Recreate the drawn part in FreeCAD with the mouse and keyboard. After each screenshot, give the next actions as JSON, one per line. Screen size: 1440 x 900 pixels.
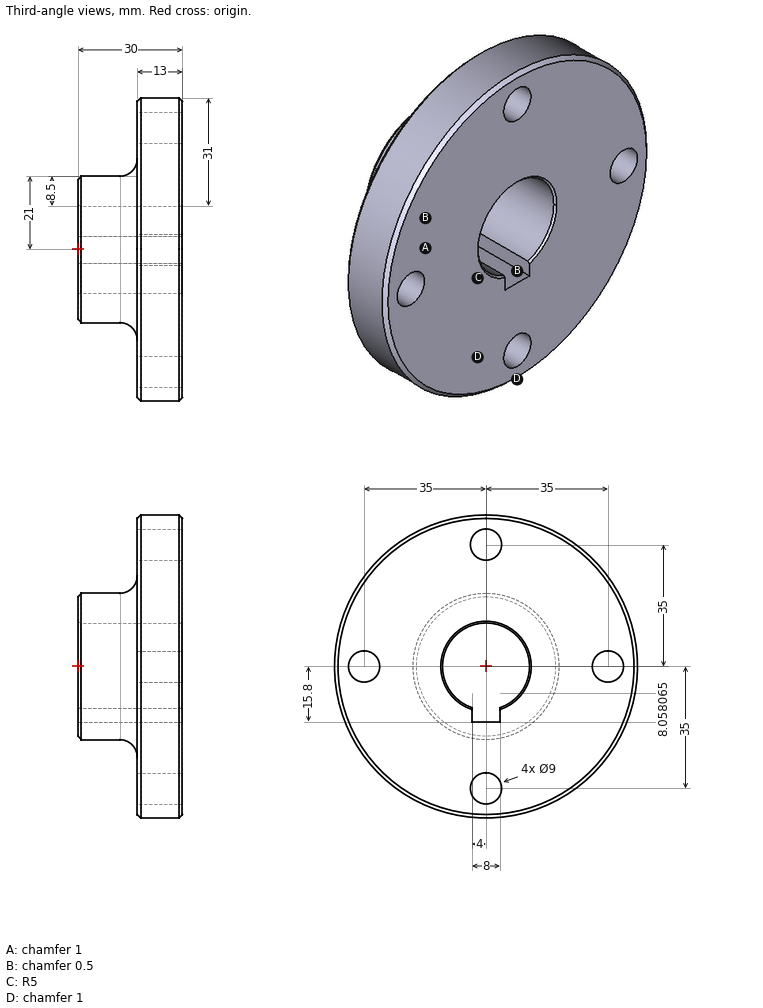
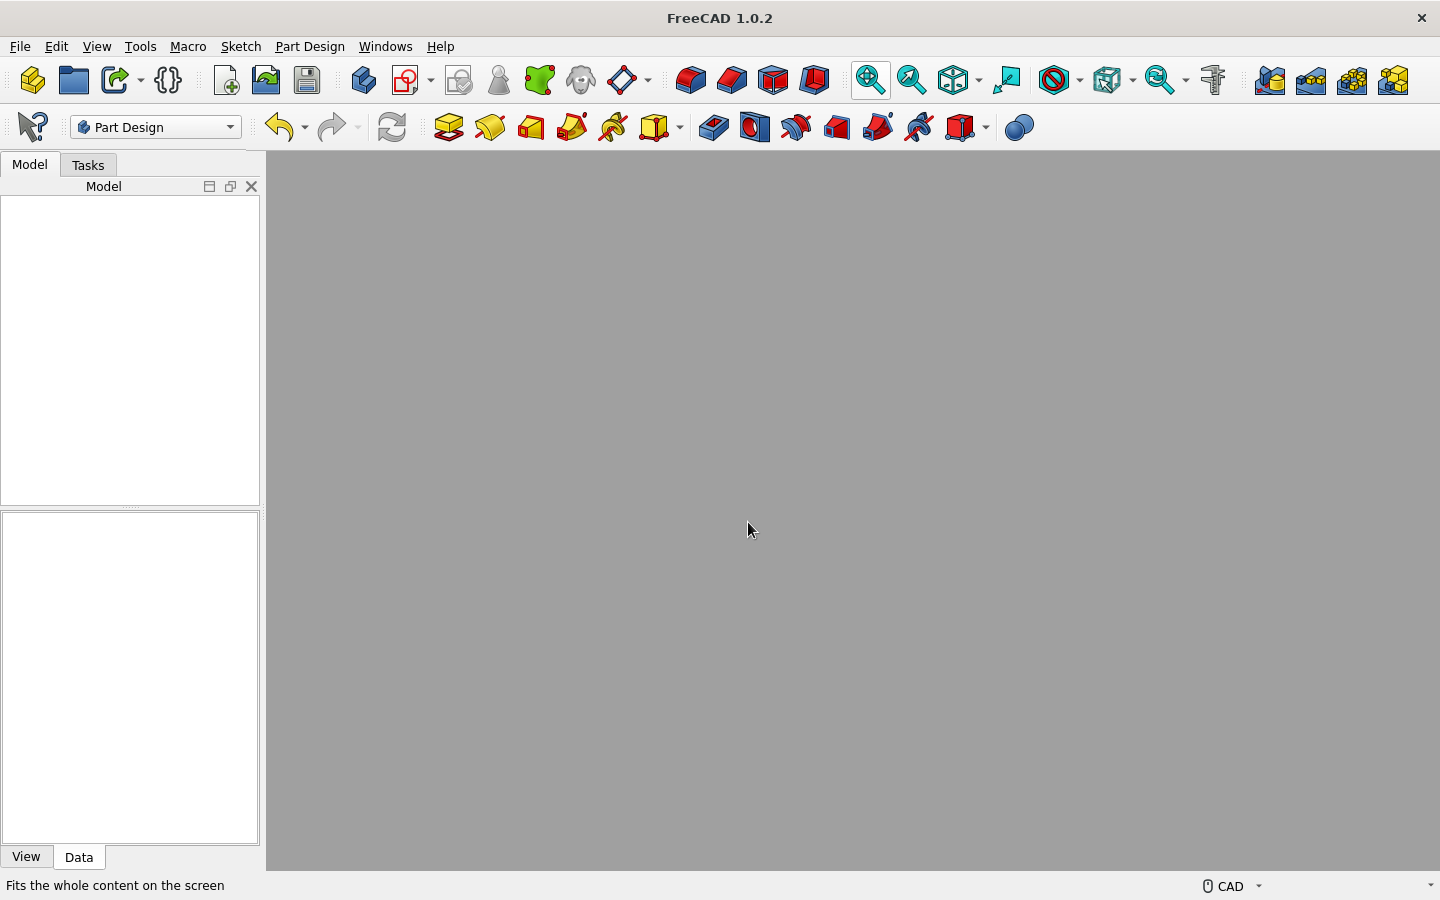
{"action": "left_click", "coordinate": [225, 80]}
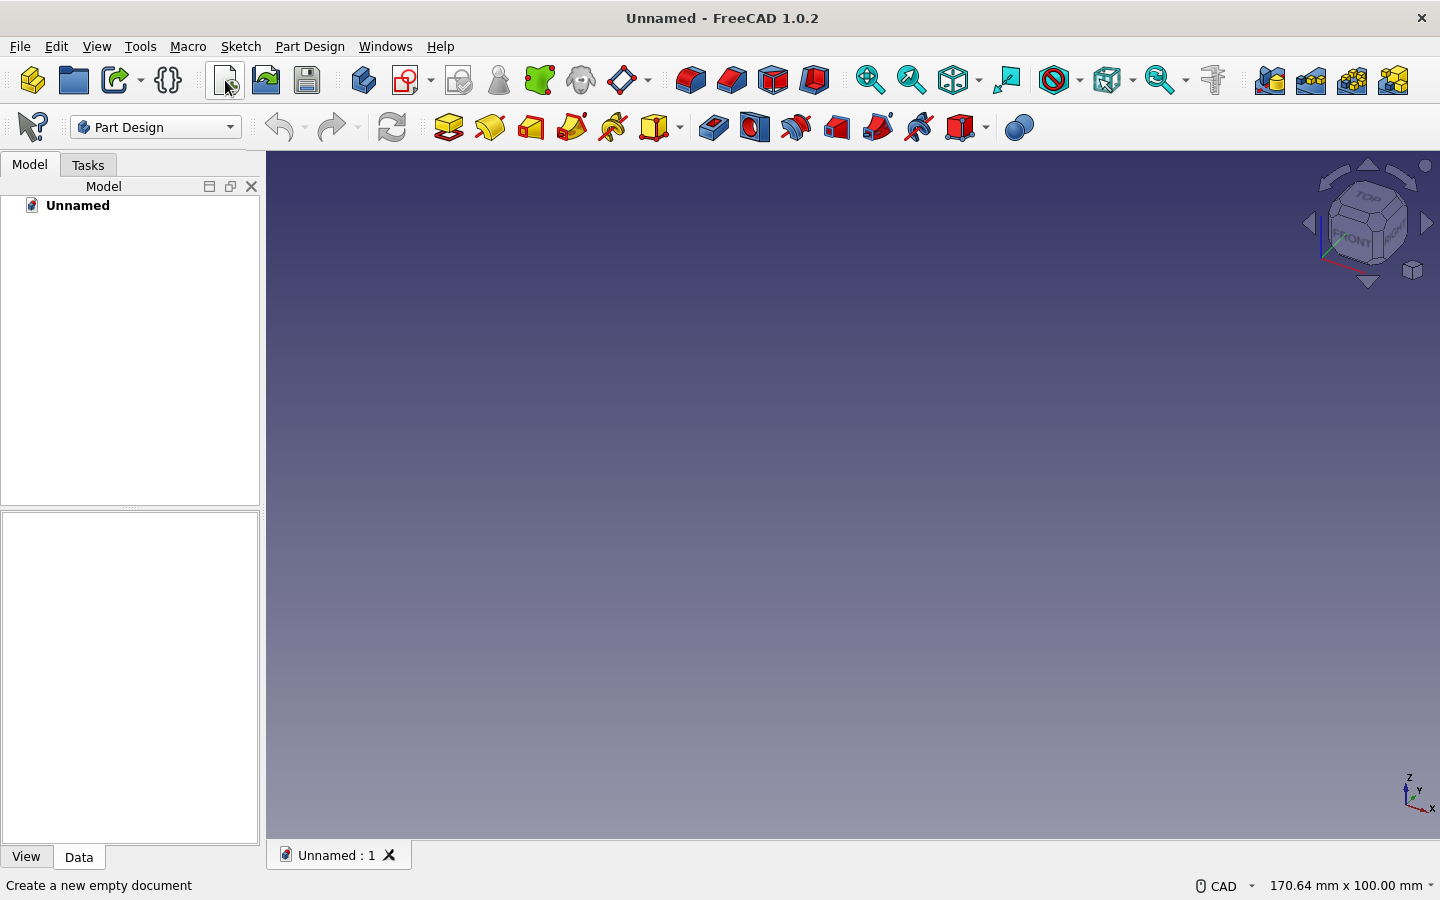
{"action": "left_click", "coordinate": [404, 80]}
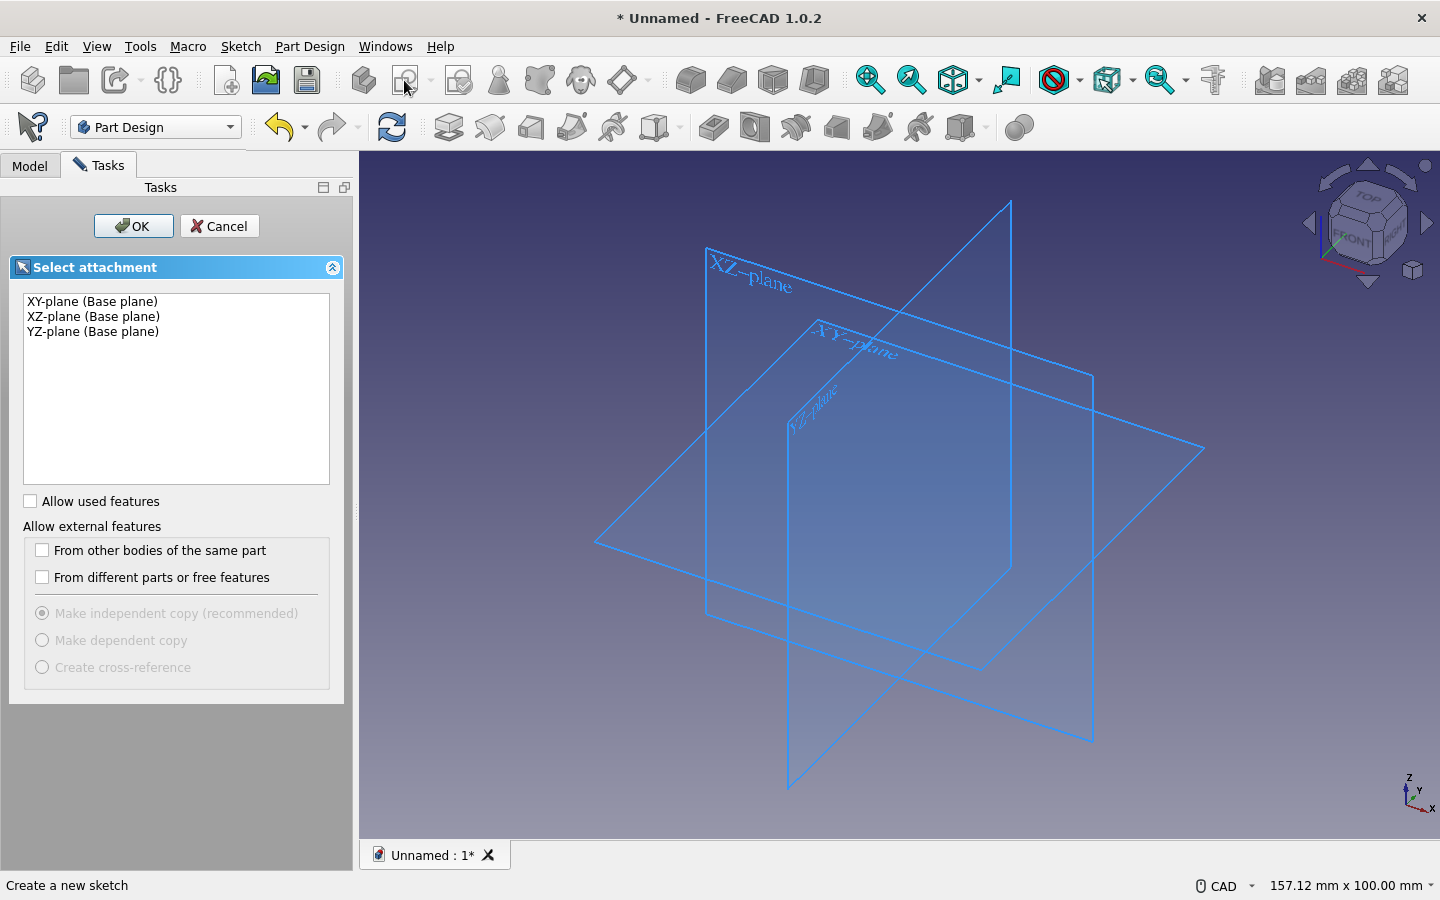
{"action": "left_click", "coordinate": [84, 302]}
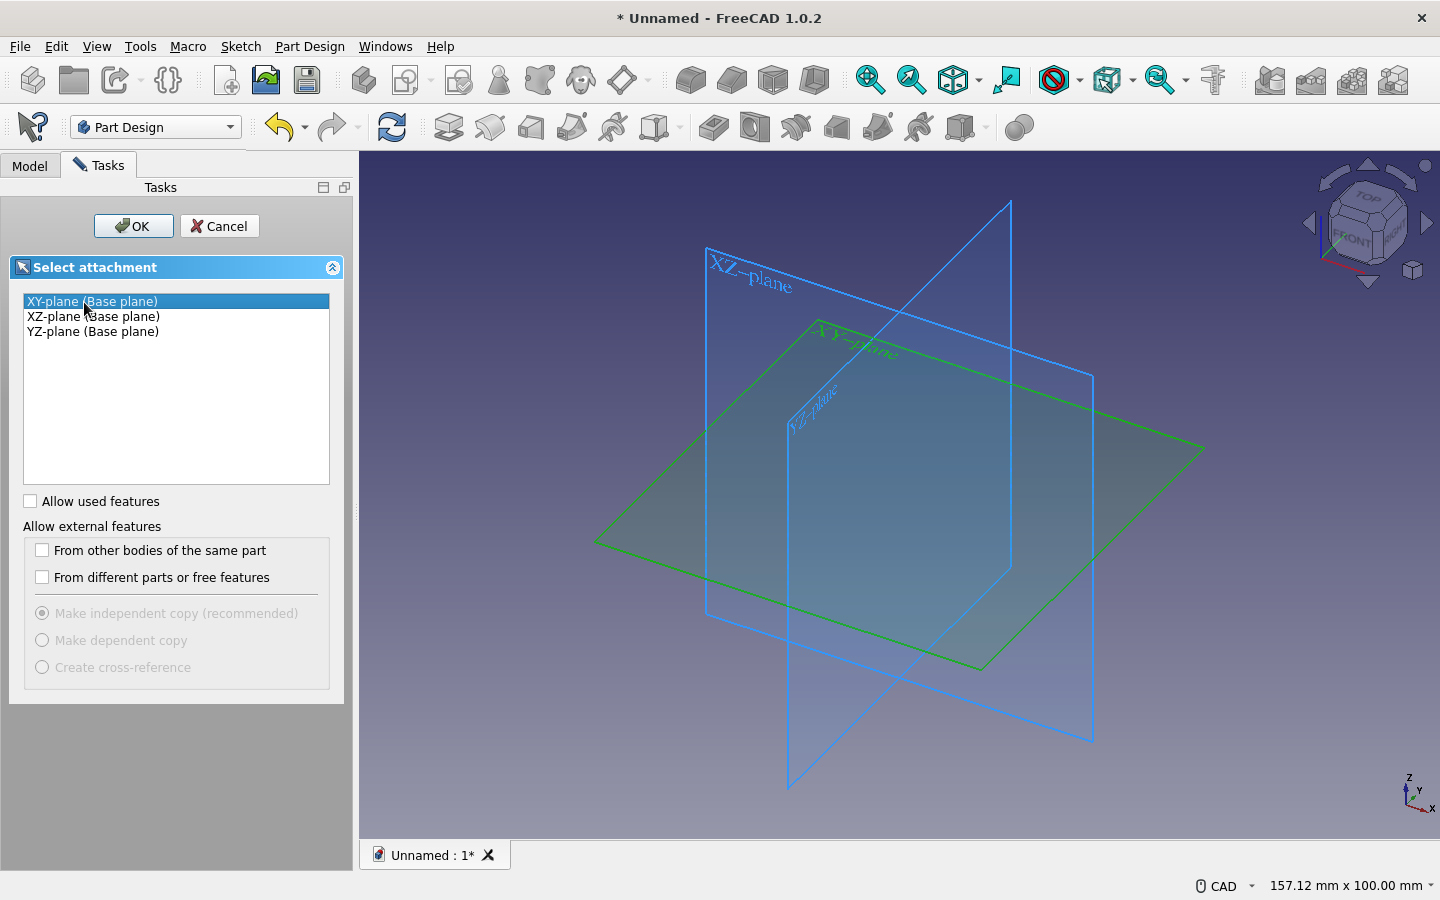
{"action": "left_click", "coordinate": [134, 226]}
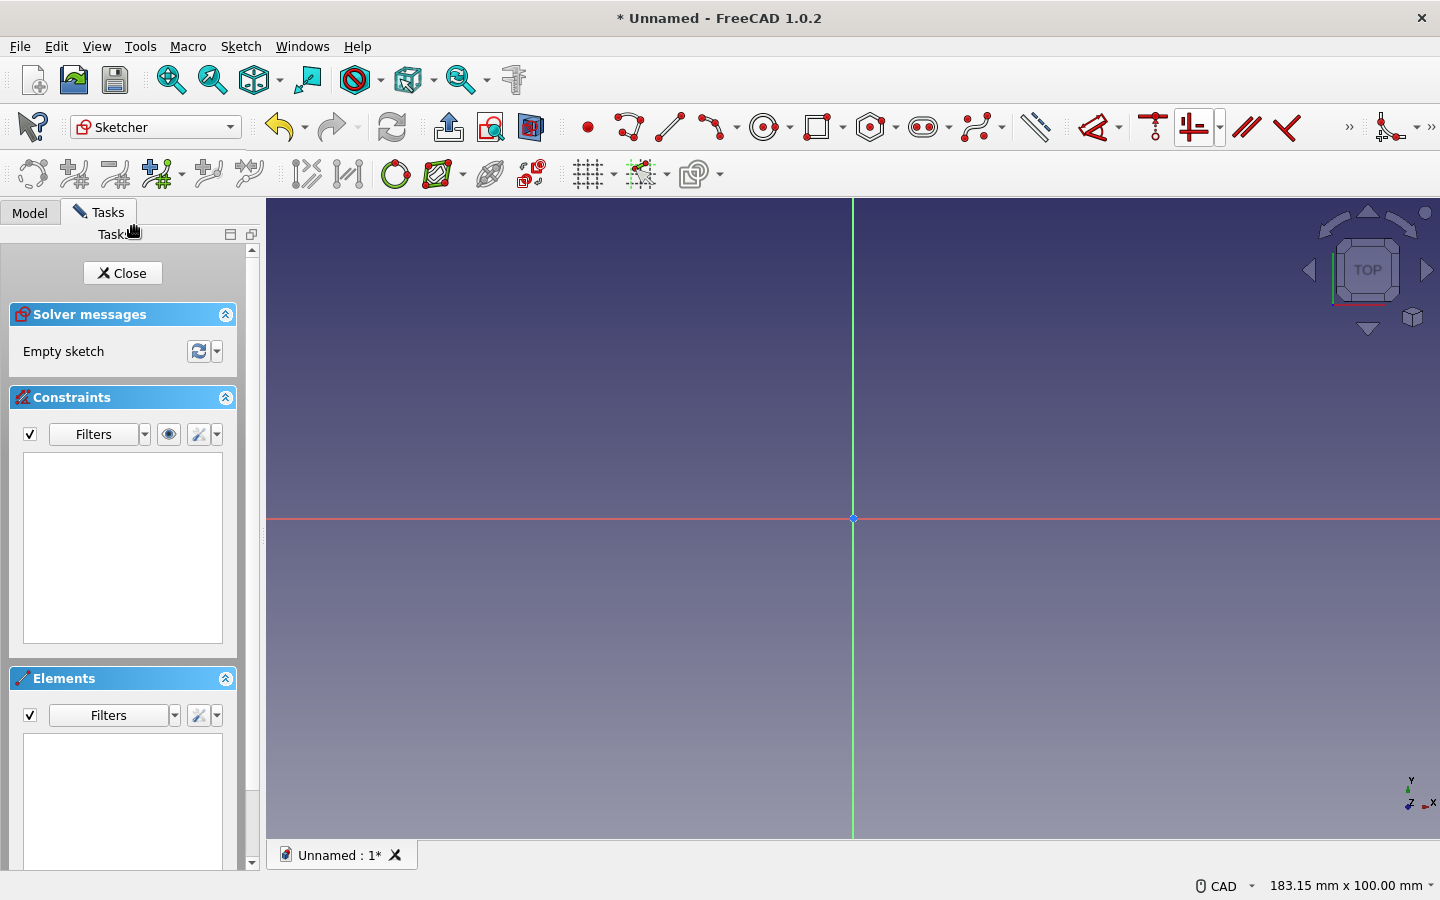
{"action": "scroll", "coordinate": [294, 811], "scroll_direction": "down", "scroll_amount": 1}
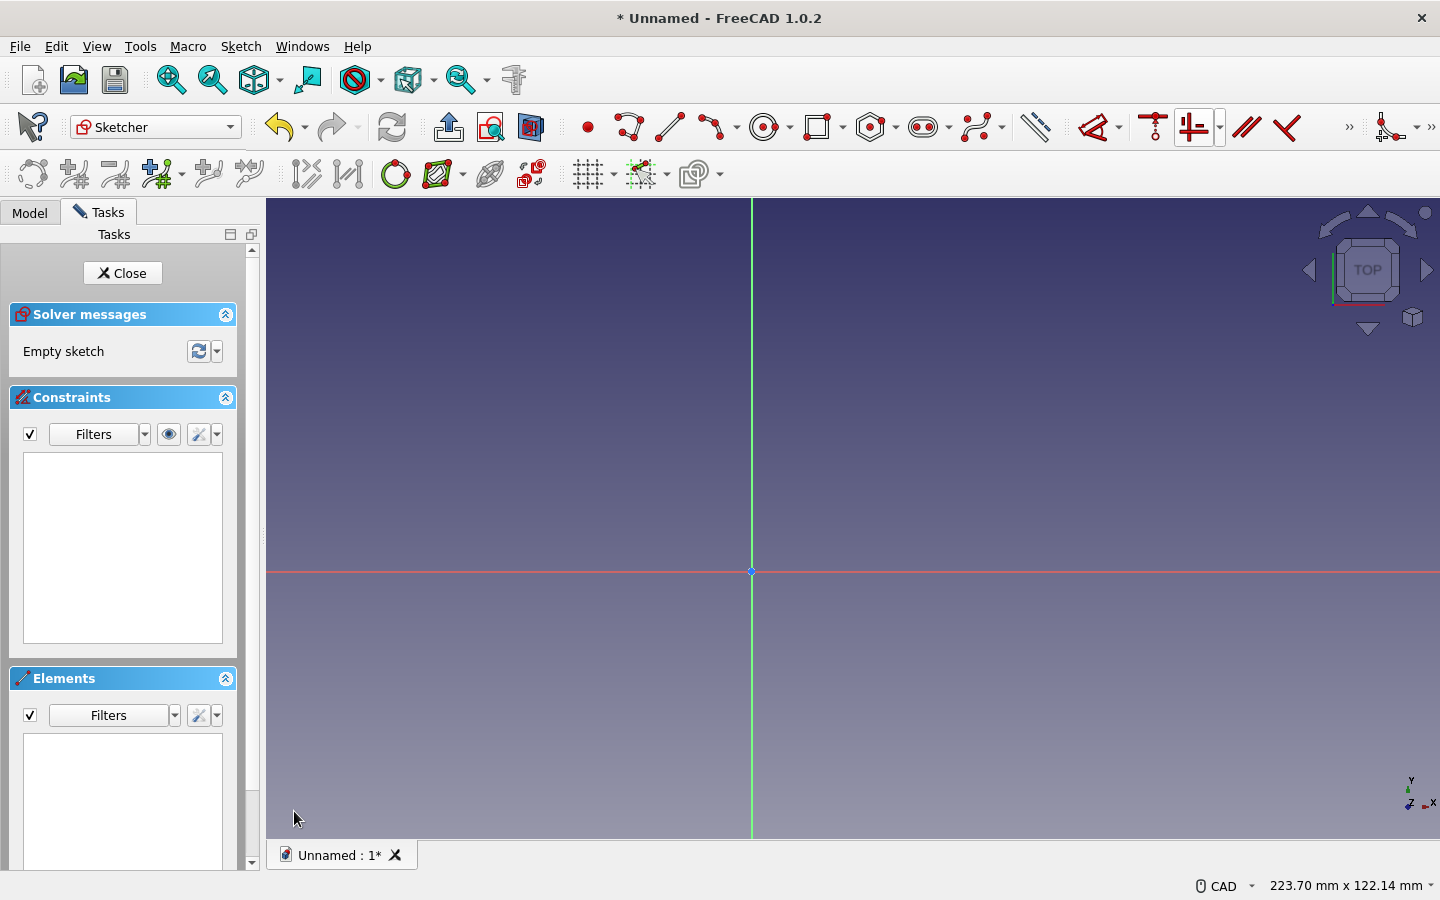
{"action": "scroll", "coordinate": [886, 383], "scroll_direction": "up", "scroll_amount": 3}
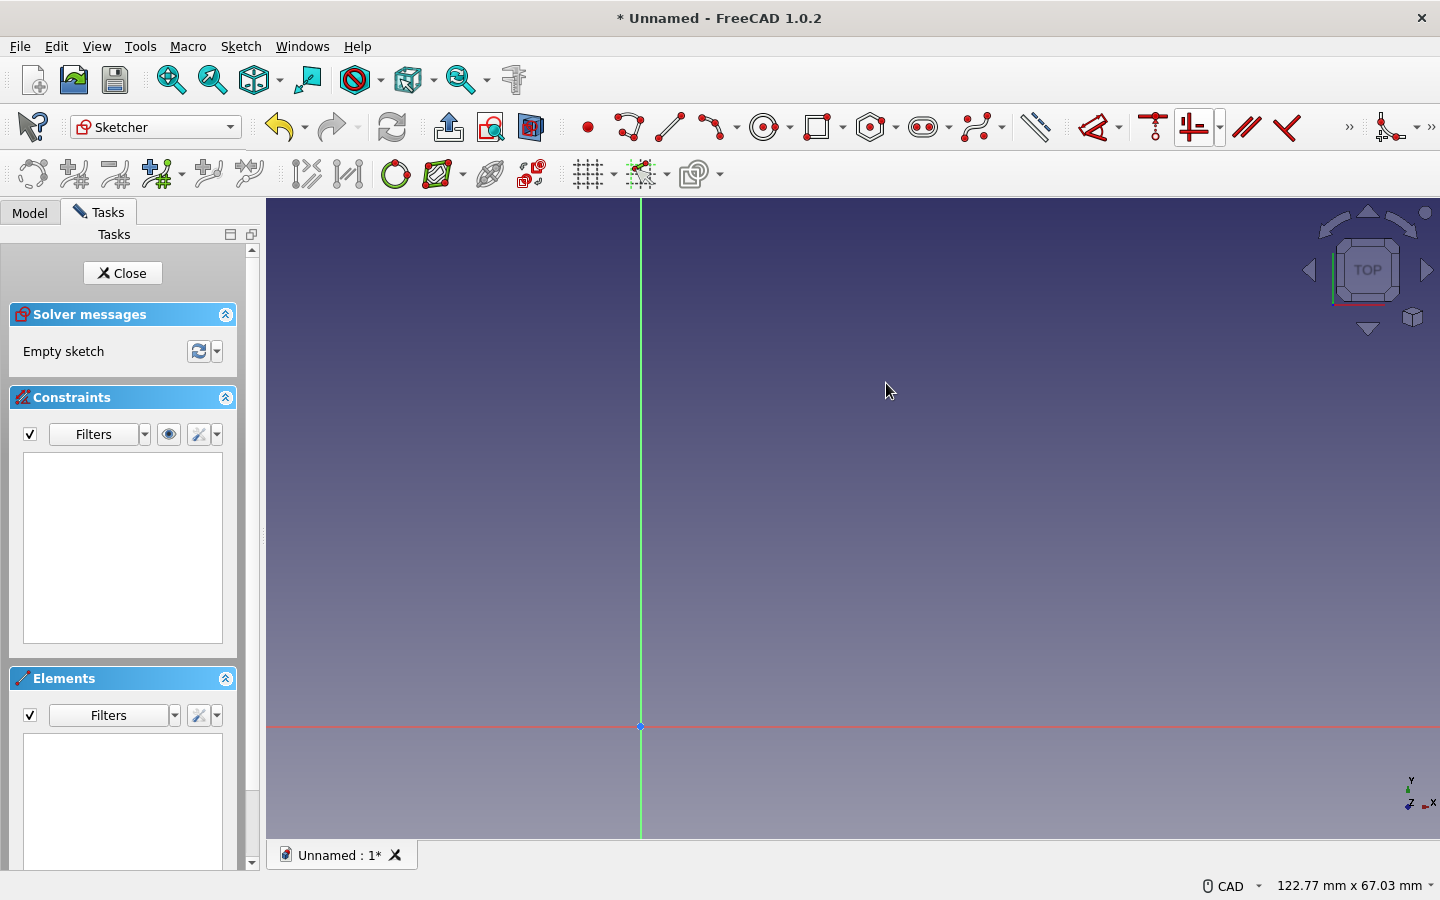
{"action": "left_click", "coordinate": [629, 128]}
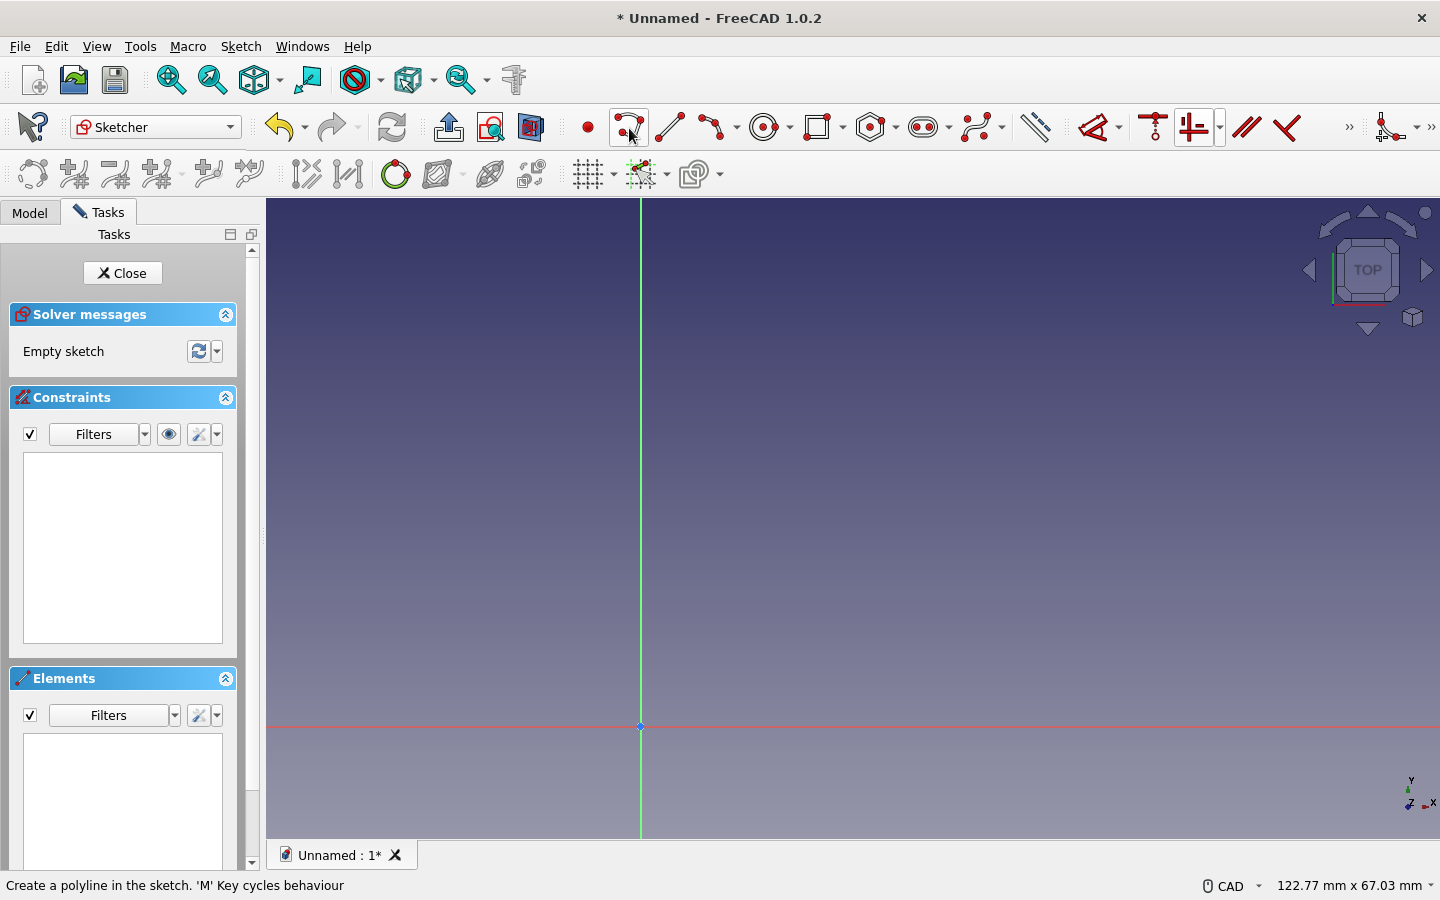
{"action": "left_click", "coordinate": [641, 607]}
{"action": "left_click", "coordinate": [928, 607]}
{"action": "left_click", "coordinate": [928, 311]}
{"action": "left_click", "coordinate": [803, 311]}
{"action": "left_click", "coordinate": [803, 526]}
{"action": "left_click", "coordinate": [650, 526]}
{"action": "left_click", "coordinate": [641, 608]}
{"action": "key", "text": "Escape"}
{"action": "key", "text": "Escape"}